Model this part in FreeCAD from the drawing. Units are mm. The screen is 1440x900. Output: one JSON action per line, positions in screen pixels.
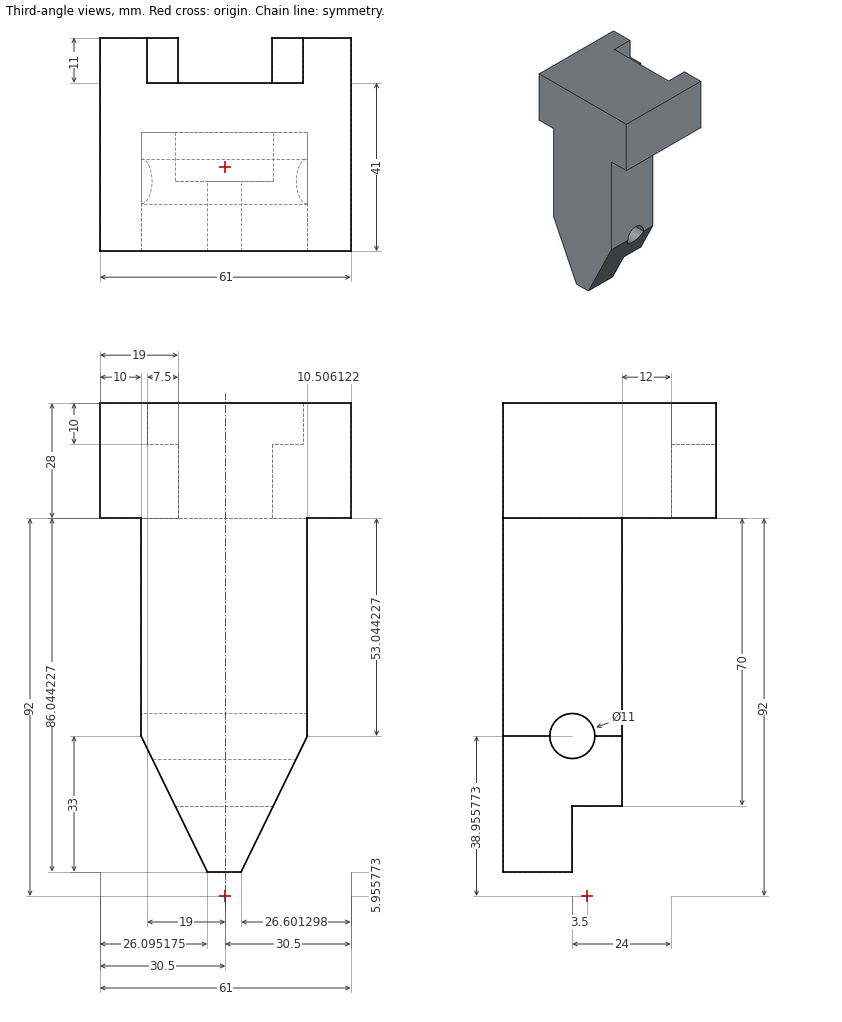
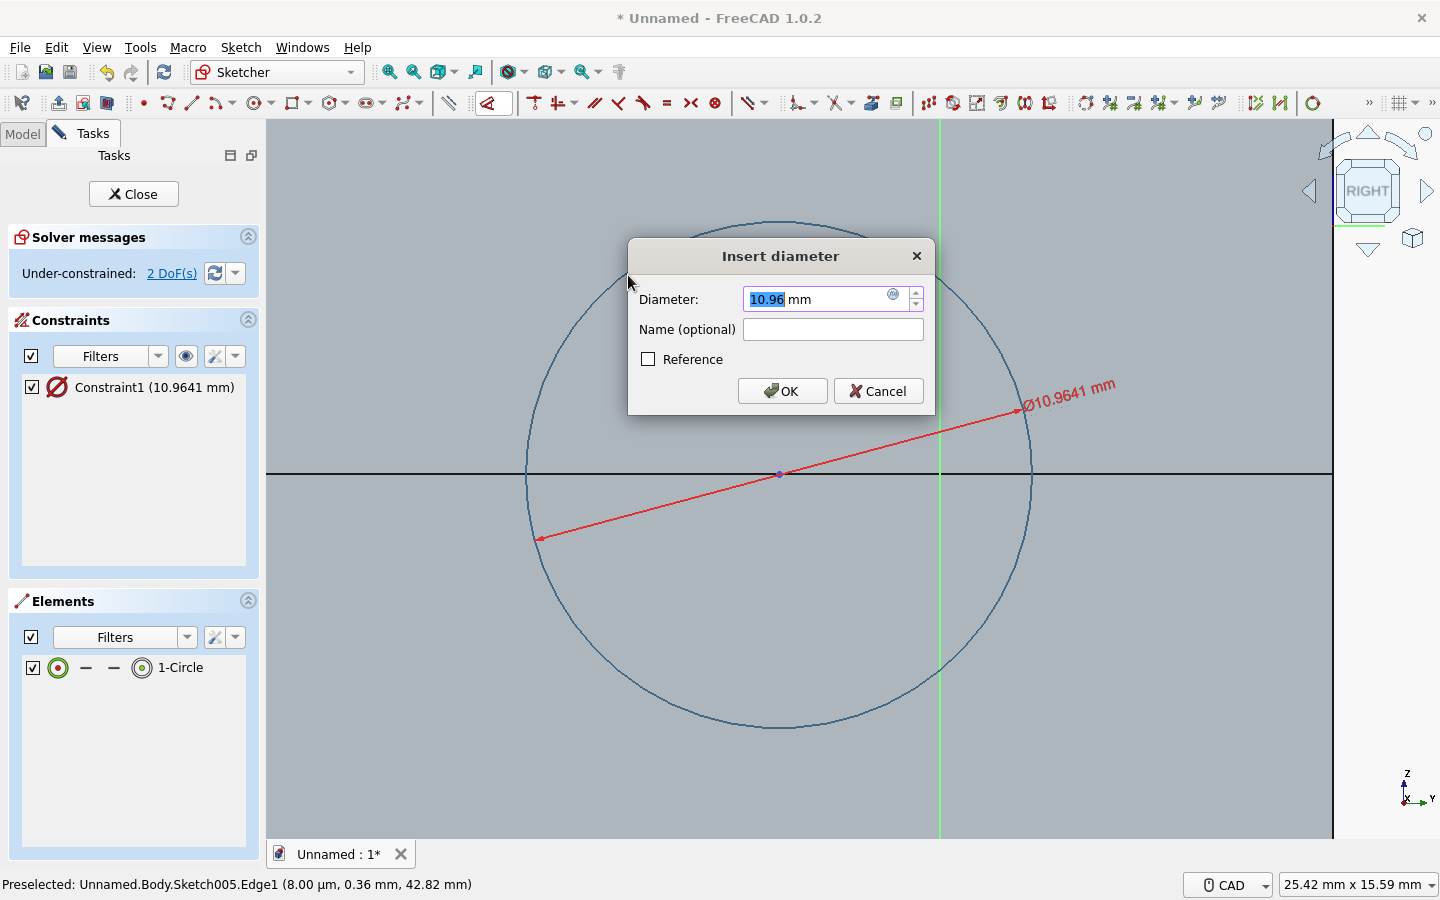
{"action": "type", "text": "11"}
{"action": "key", "text": "Return"}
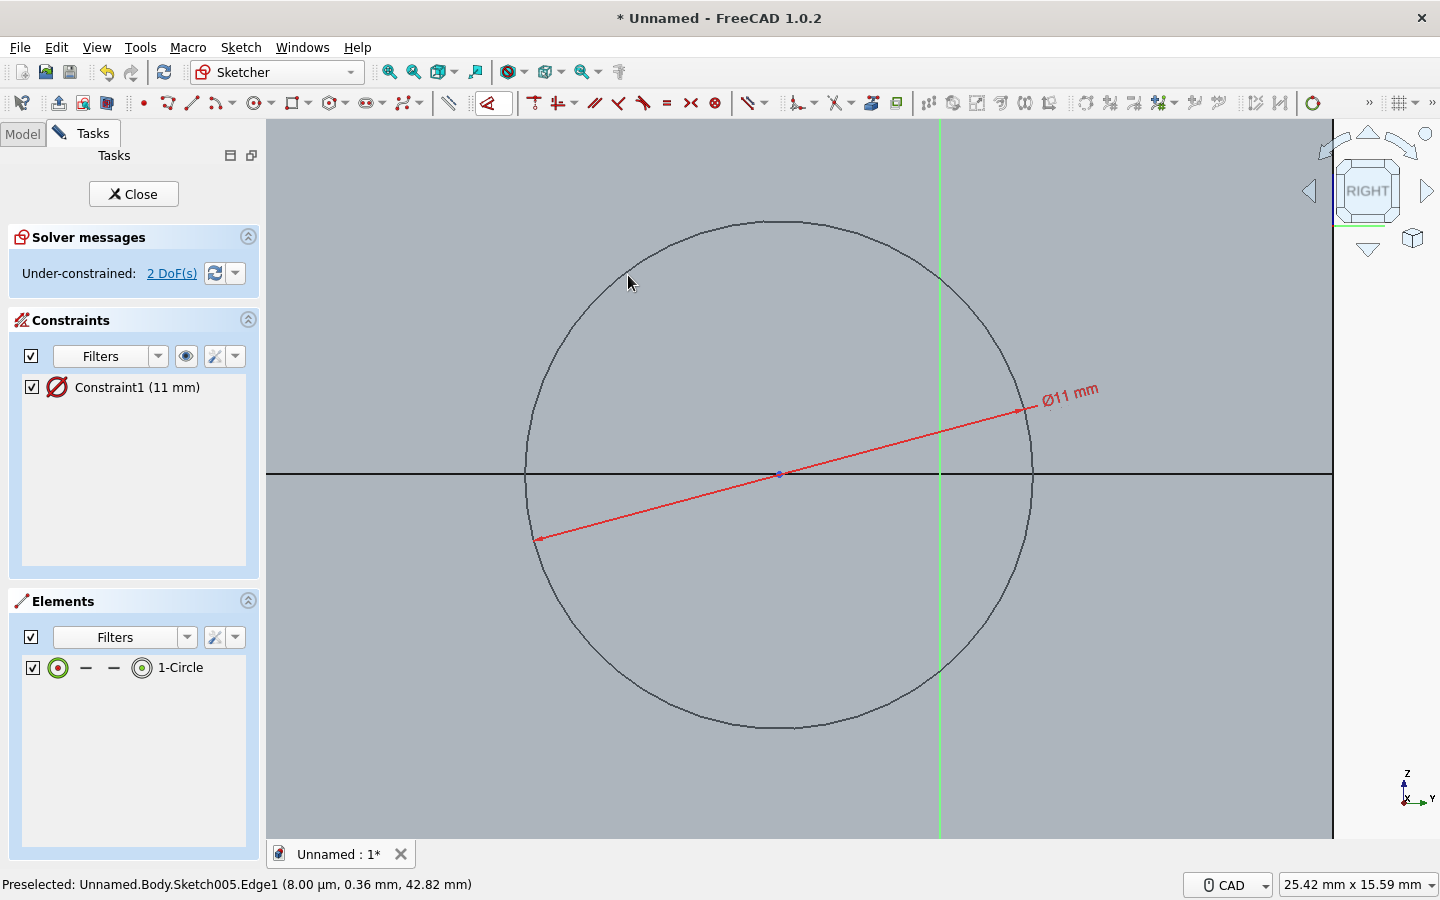
{"action": "left_click", "coordinate": [779, 475]}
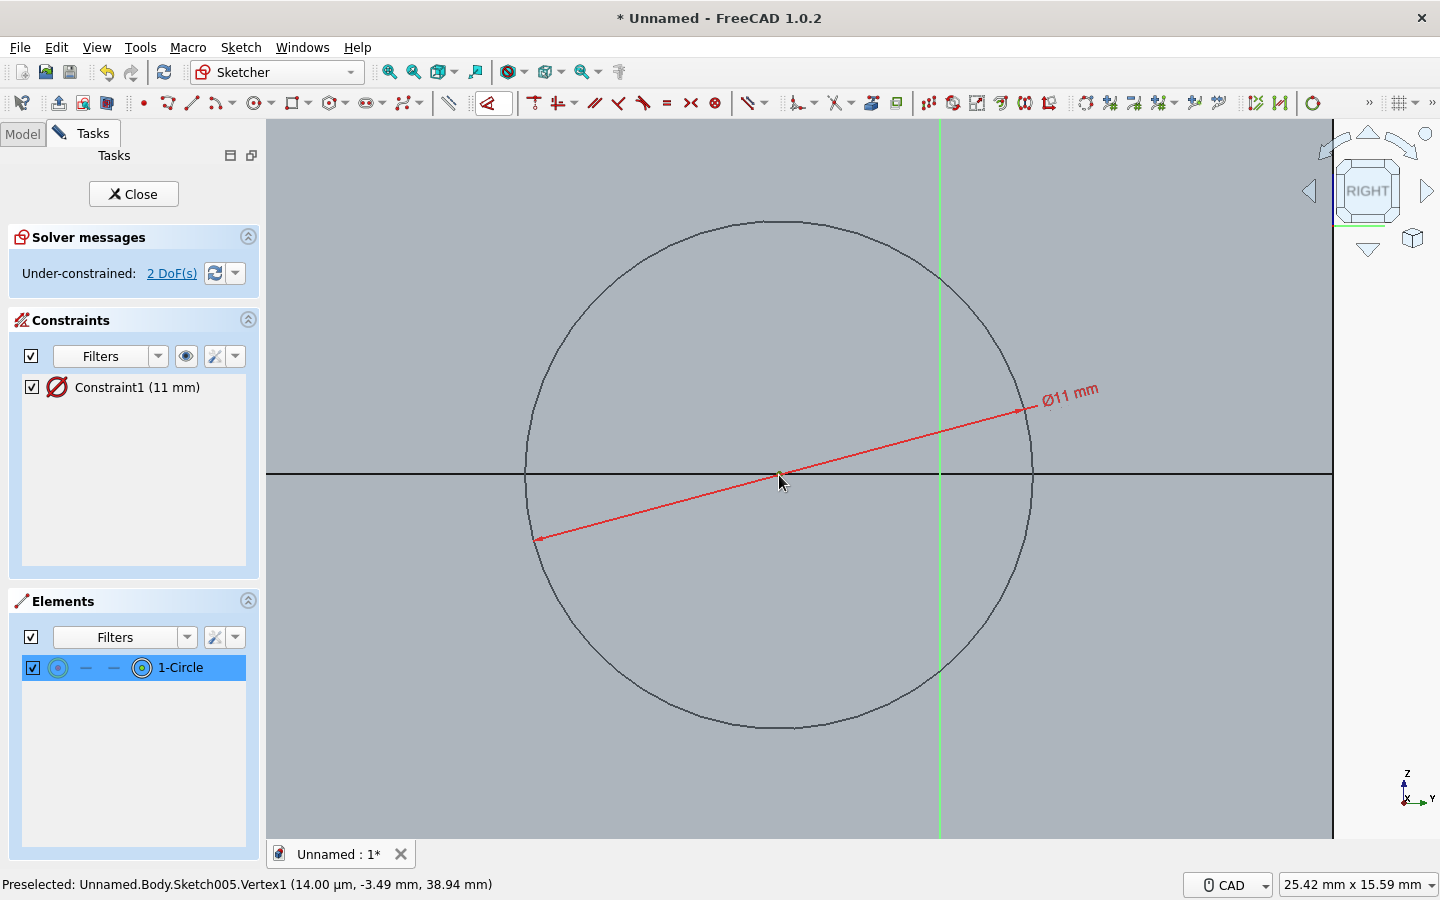
{"action": "left_click", "coordinate": [506, 104]}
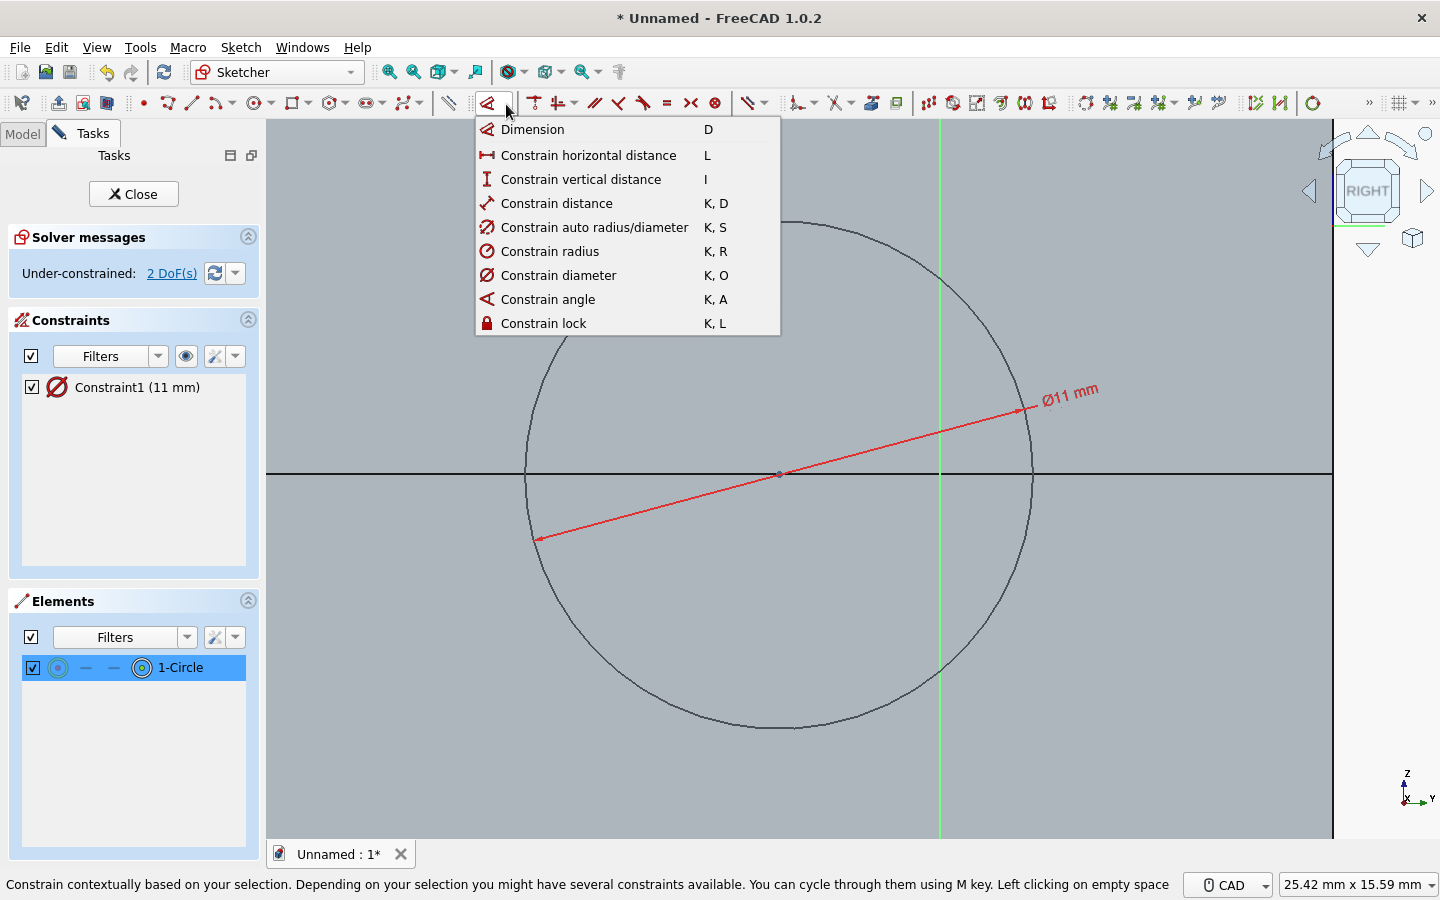
{"action": "left_click", "coordinate": [628, 155]}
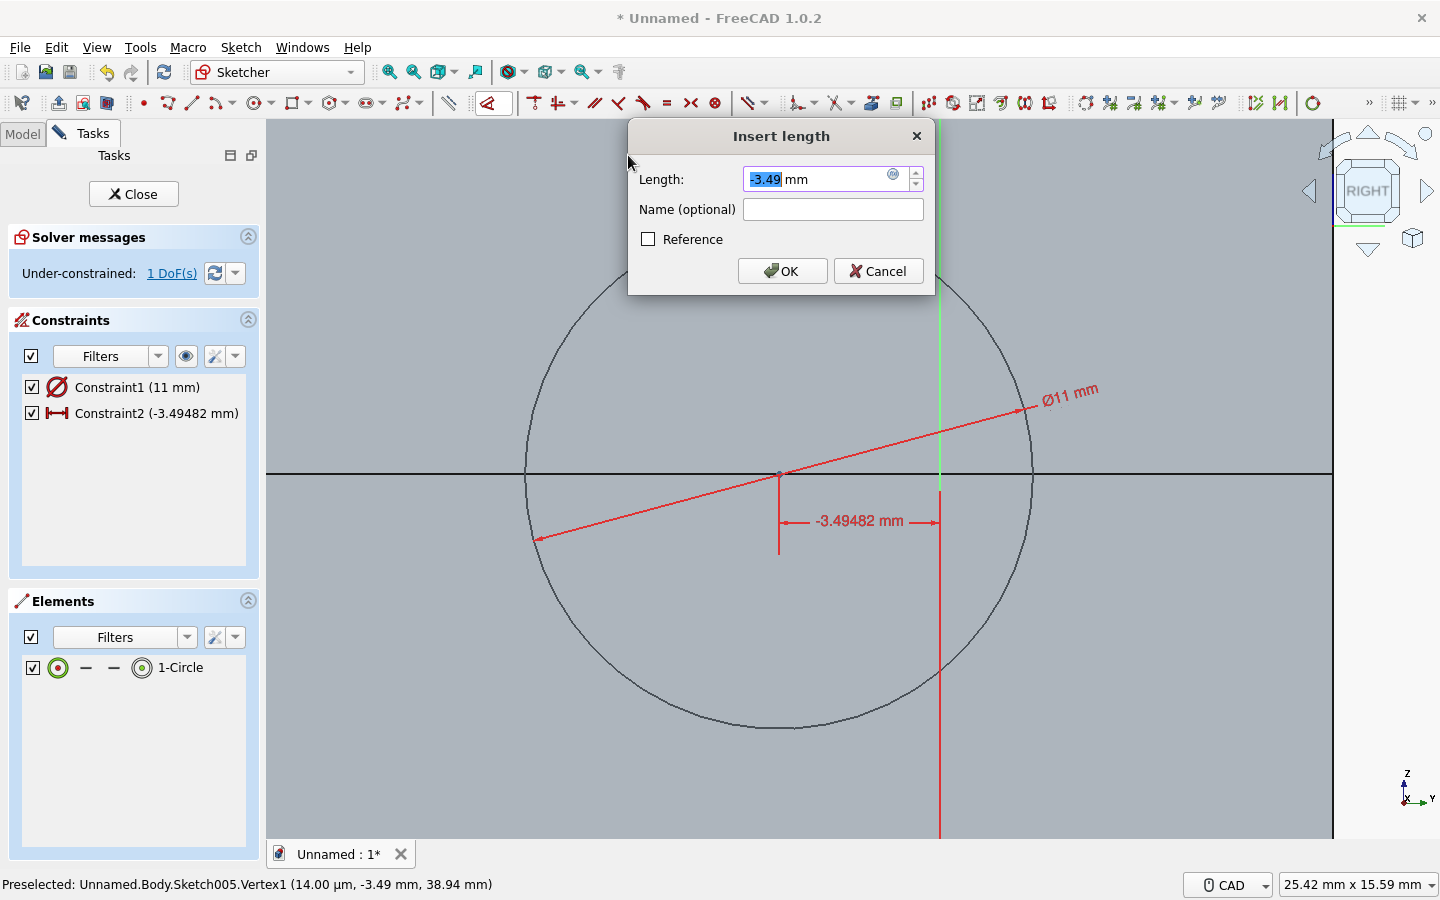
{"action": "type", "text": "-3.5"}
{"action": "key", "text": "Return"}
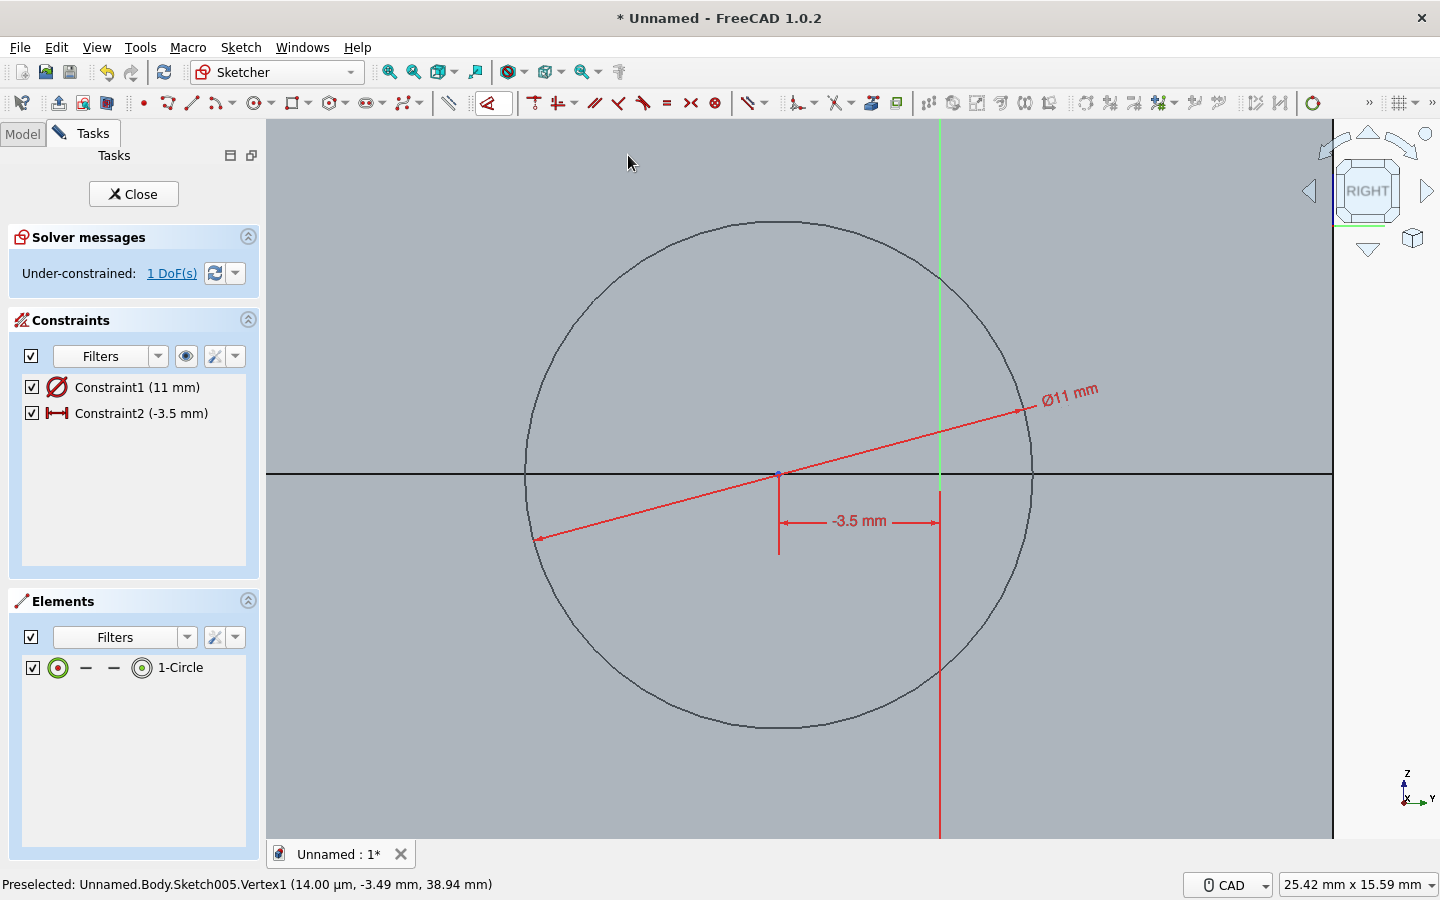
{"action": "left_click", "coordinate": [779, 475]}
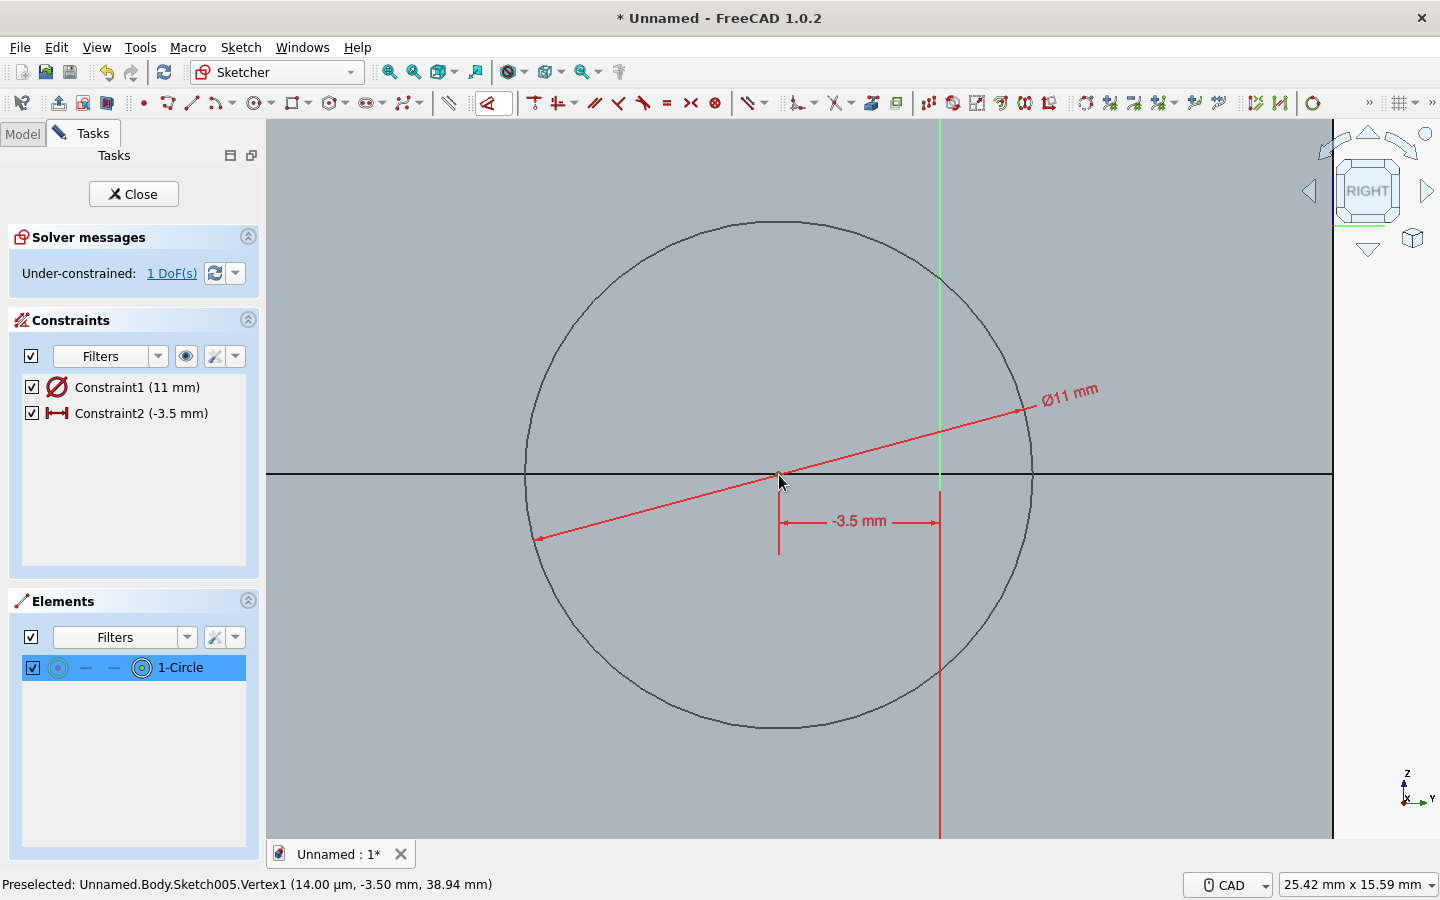
{"action": "left_click", "coordinate": [506, 104]}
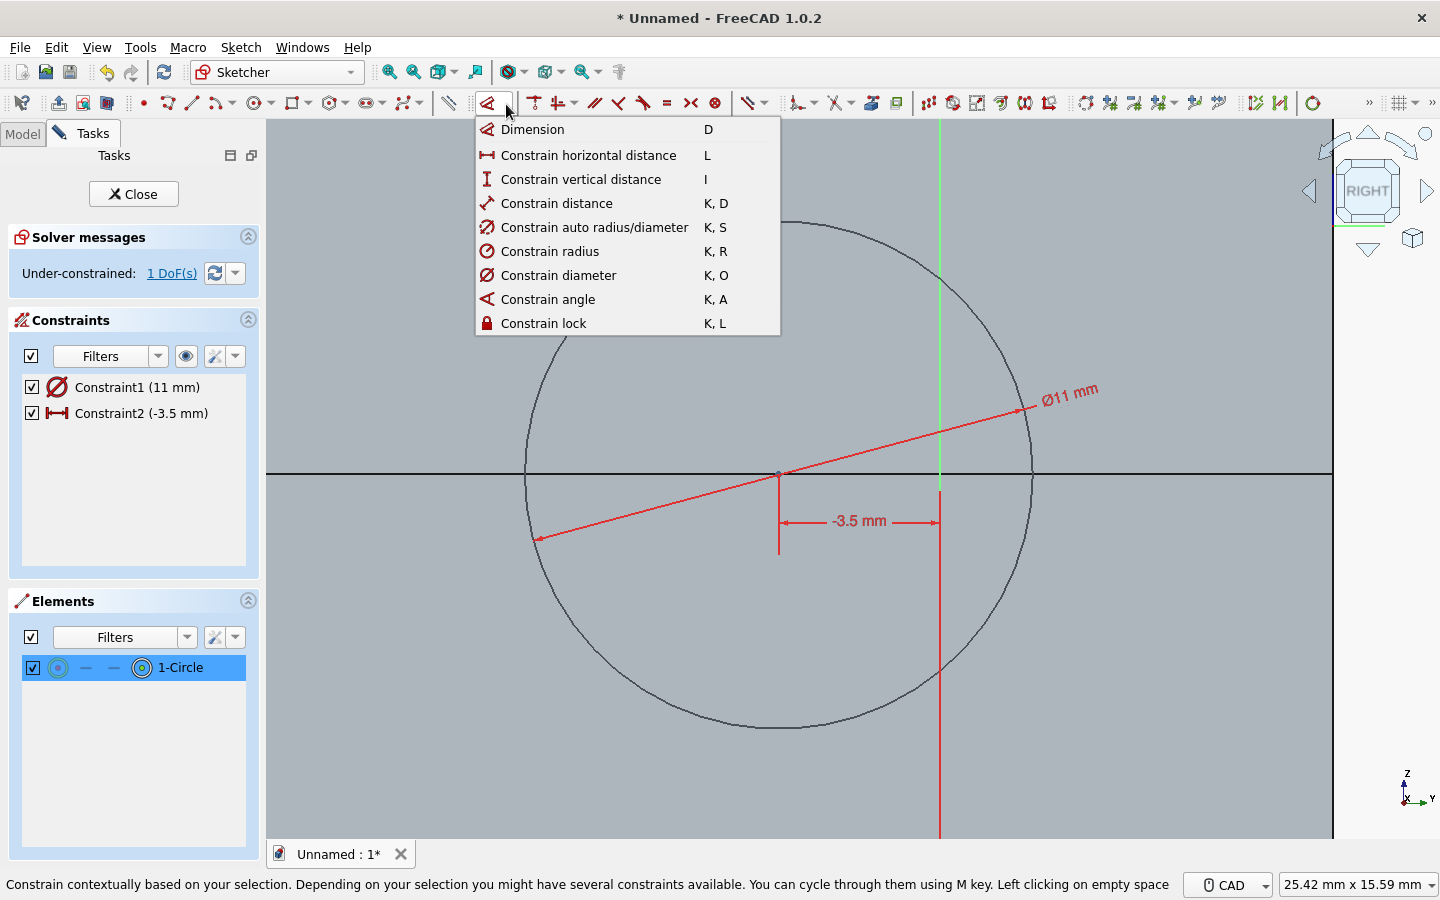
{"action": "left_click", "coordinate": [628, 179]}